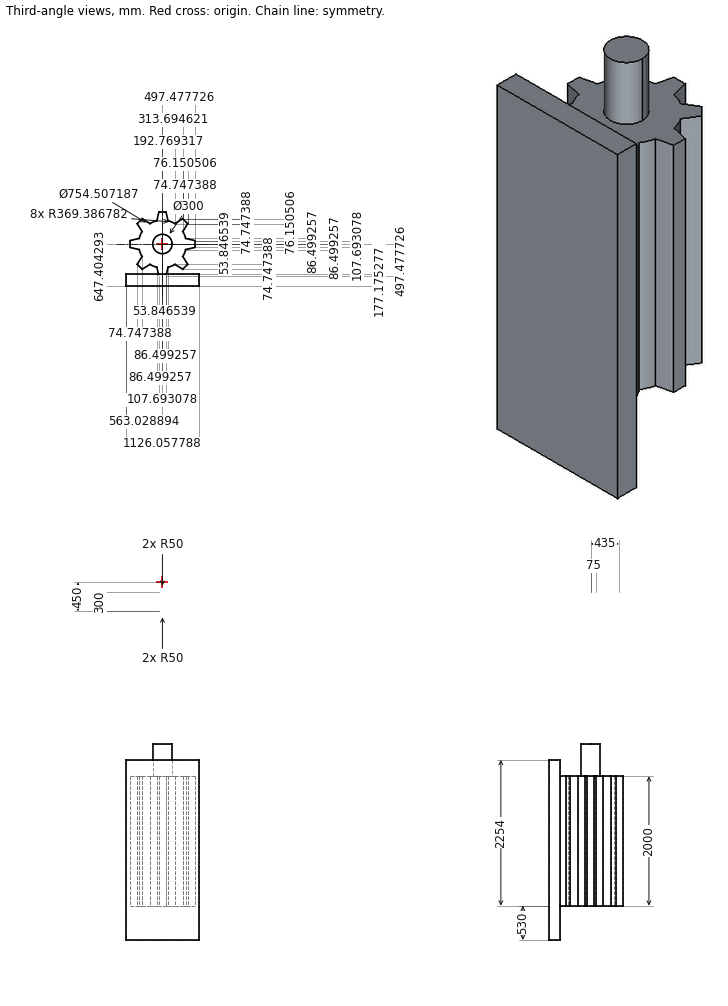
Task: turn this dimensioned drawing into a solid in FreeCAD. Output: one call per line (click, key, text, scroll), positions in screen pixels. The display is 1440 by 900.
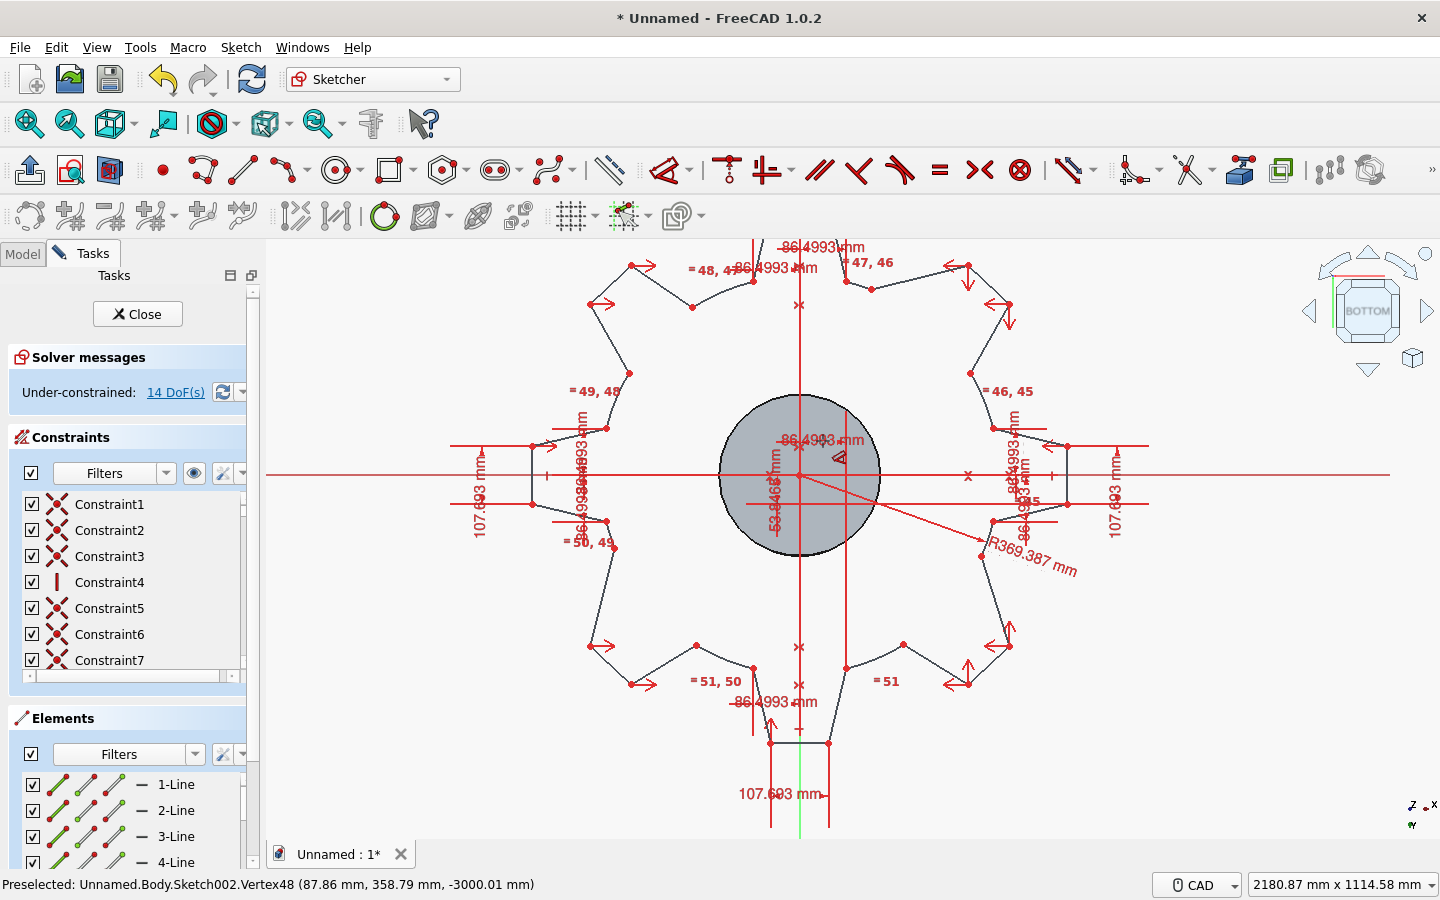
click(923, 657)
click(1002, 674)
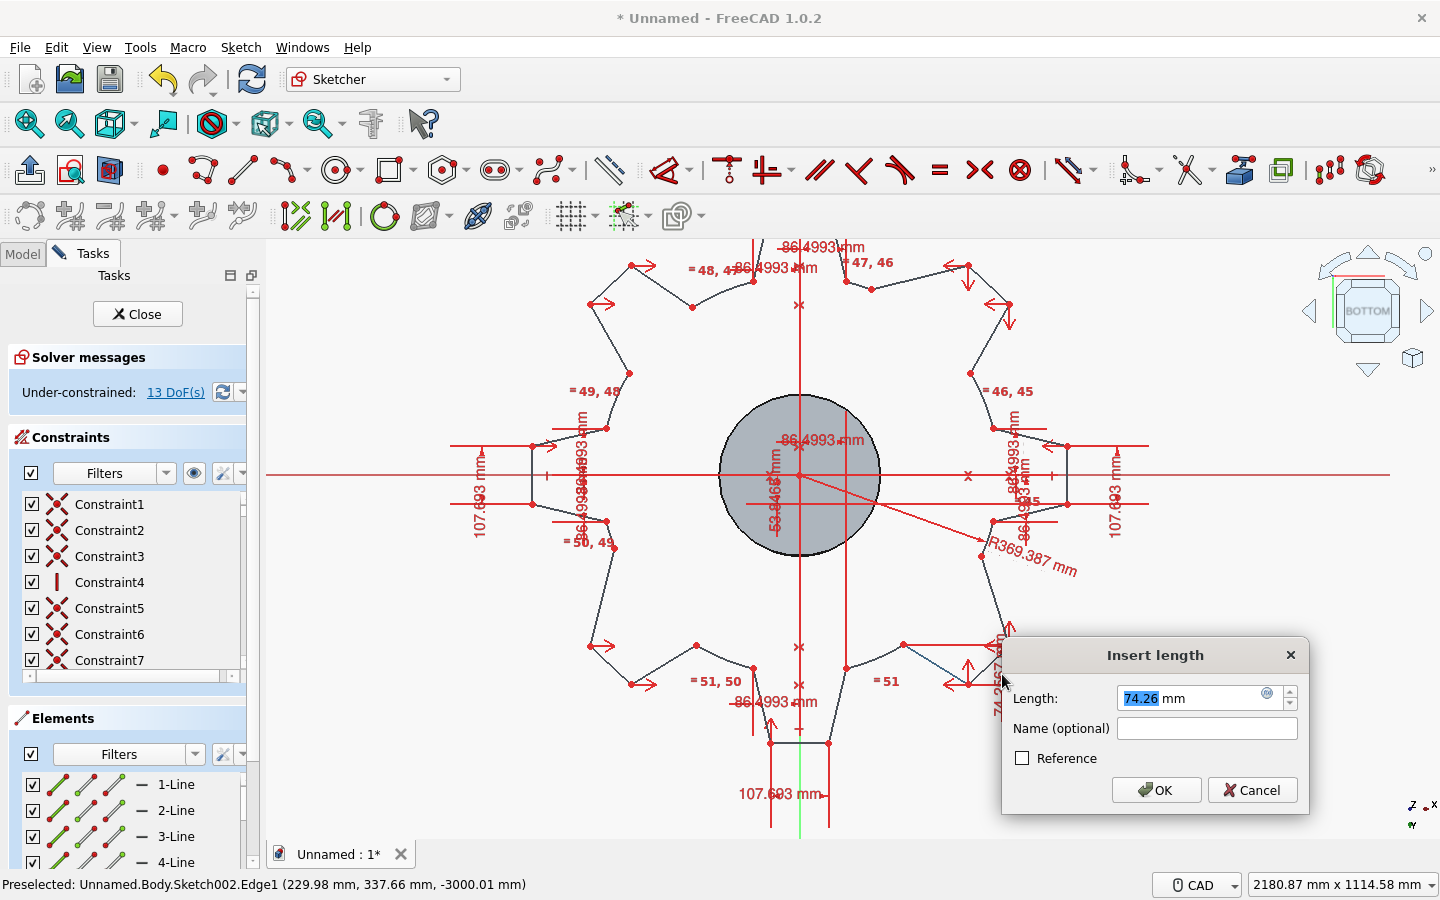
text(74.747388)
key(Return)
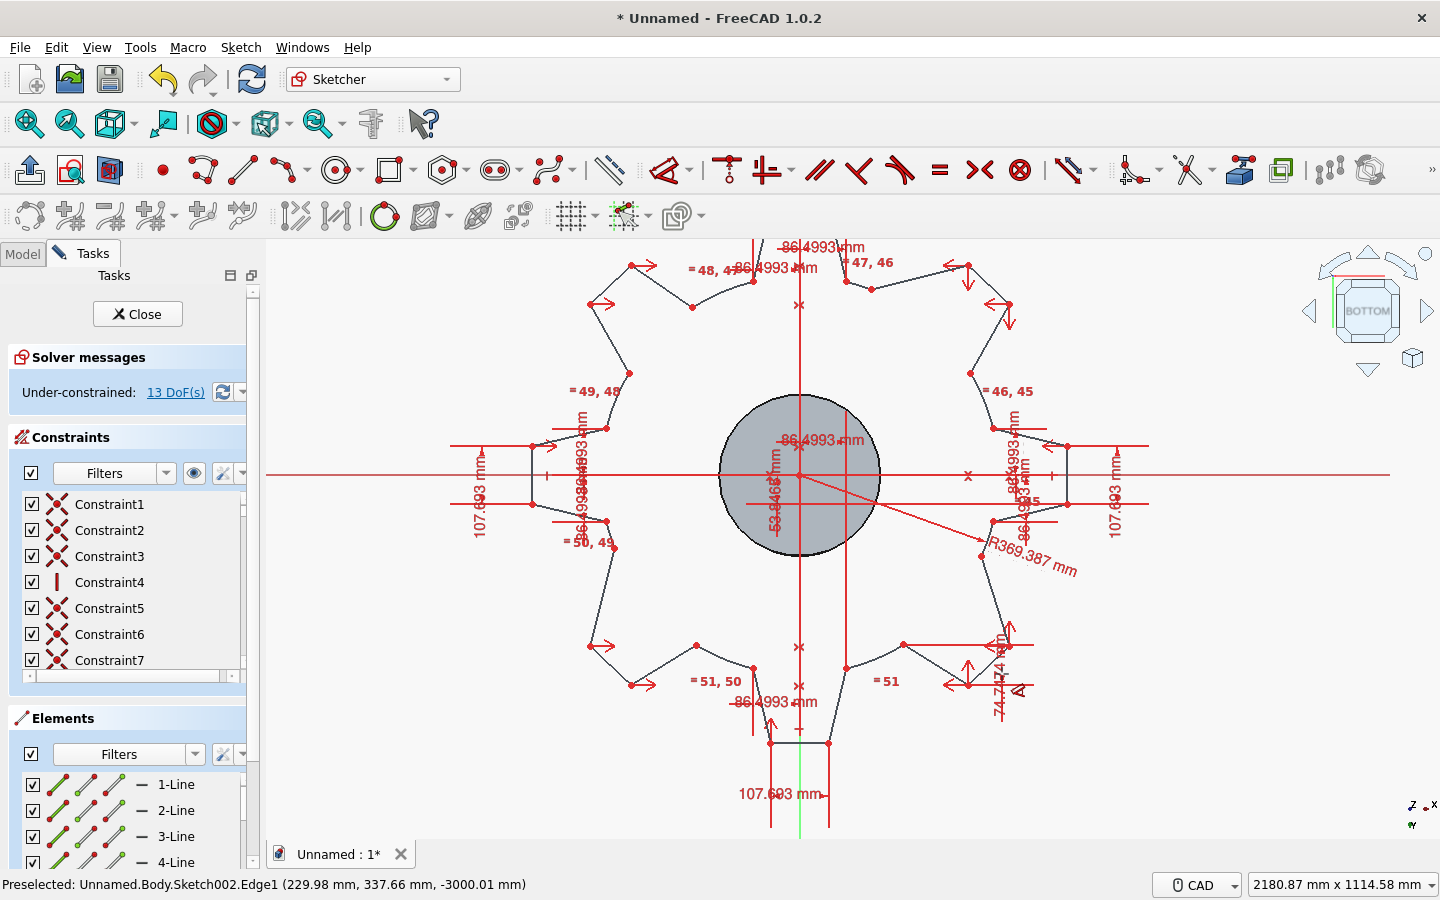
click(981, 673)
click(989, 719)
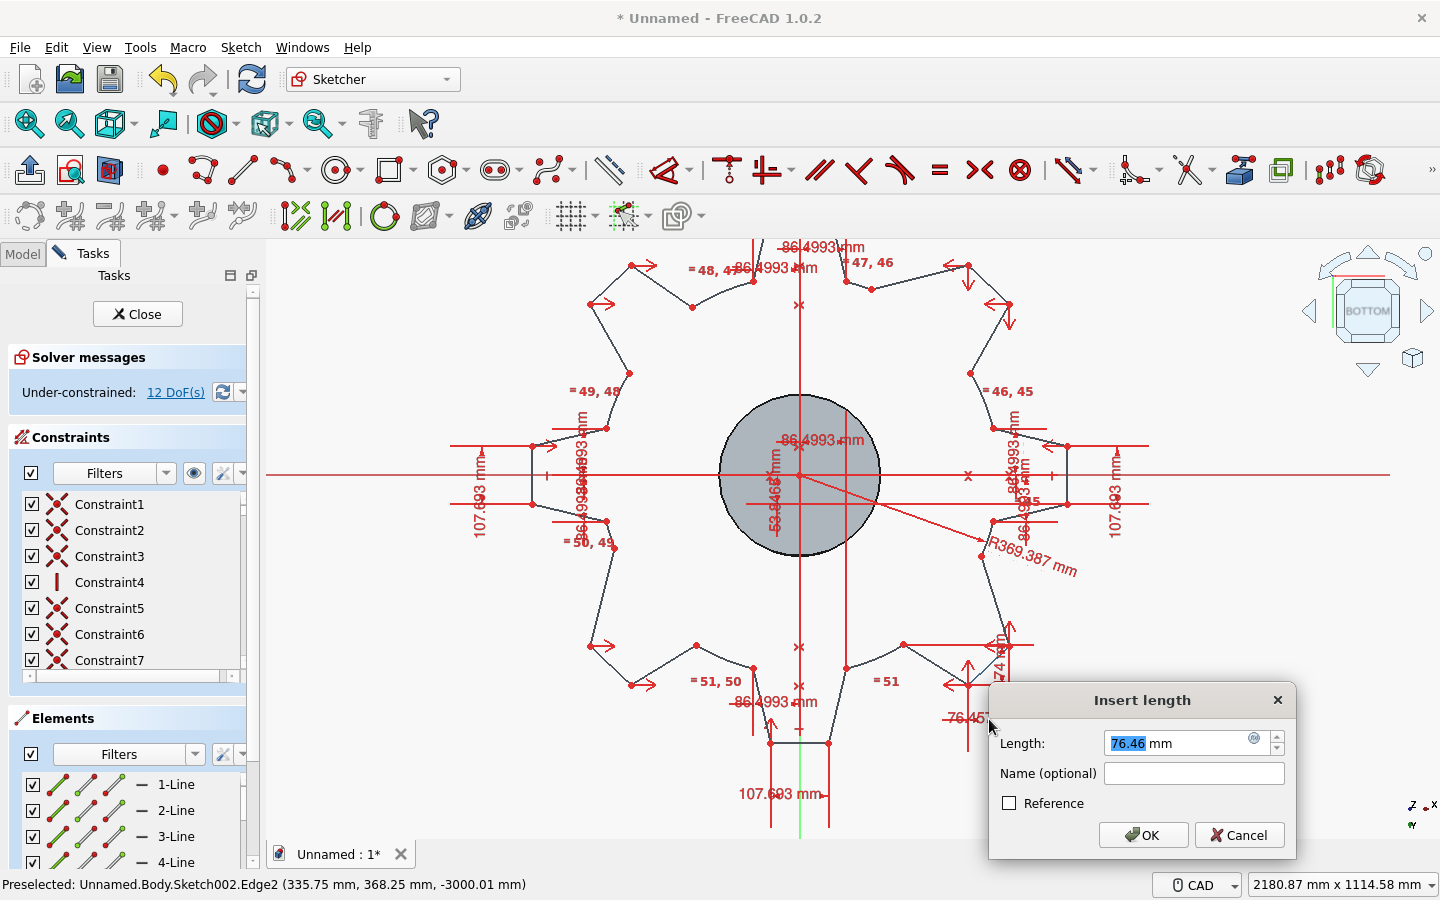
text(76.150506)
key(Return)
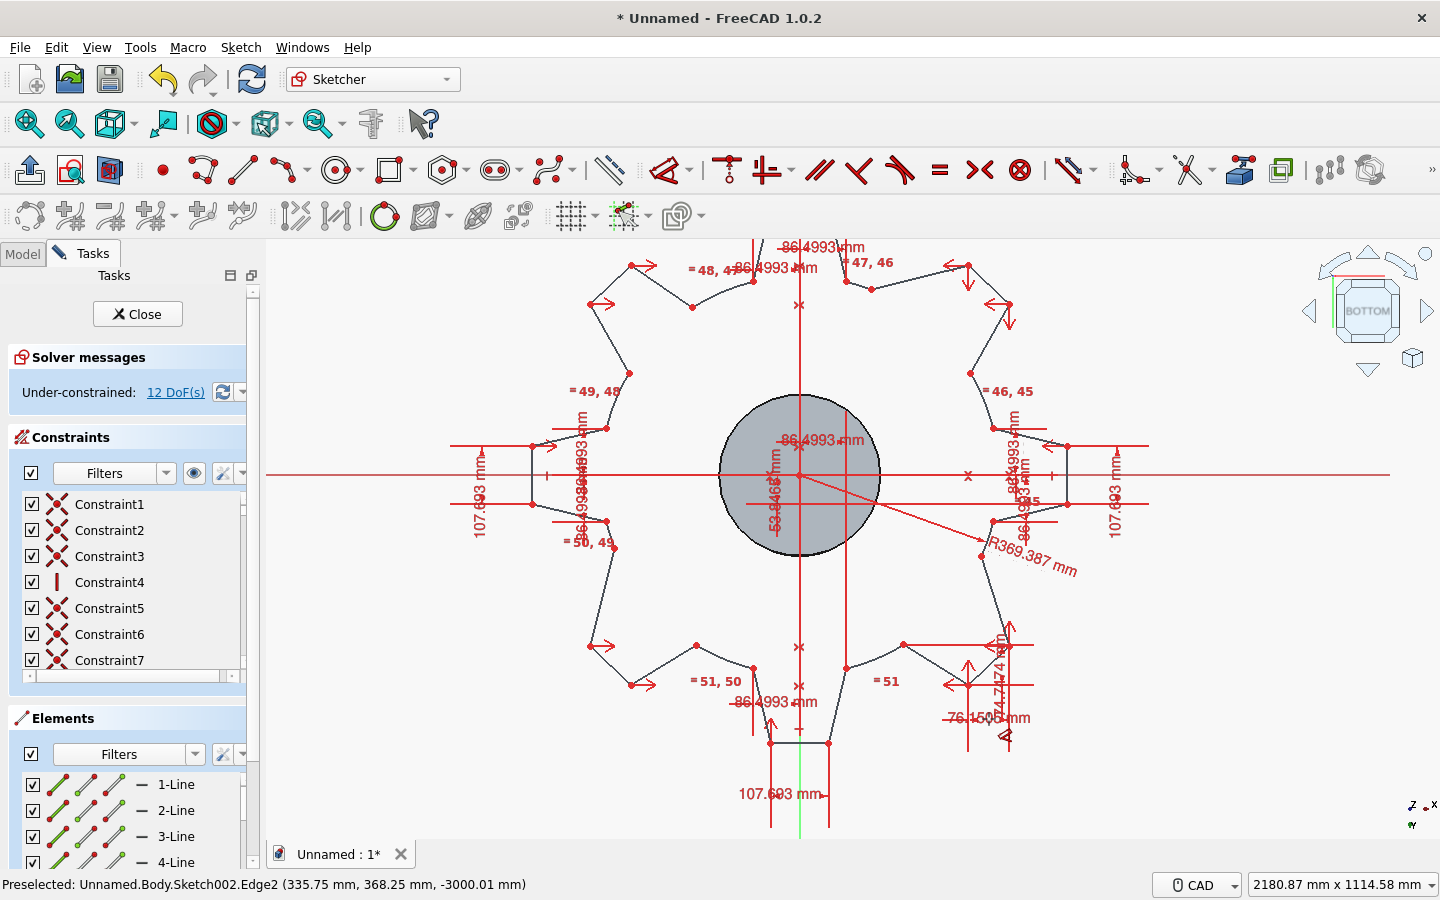
click(981, 673)
click(1043, 652)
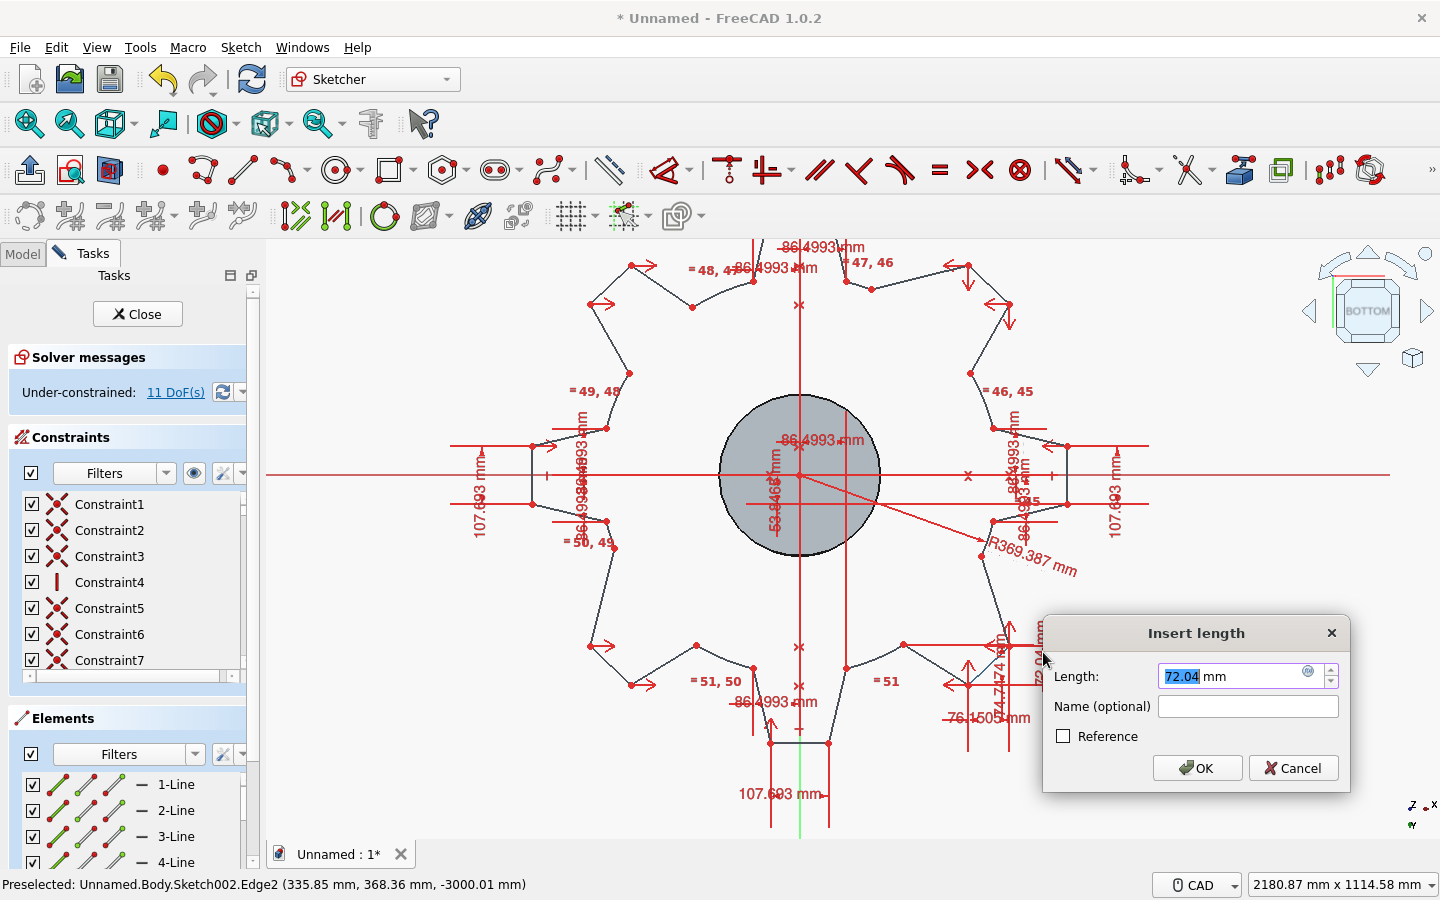
text(76.150506)
key(Return)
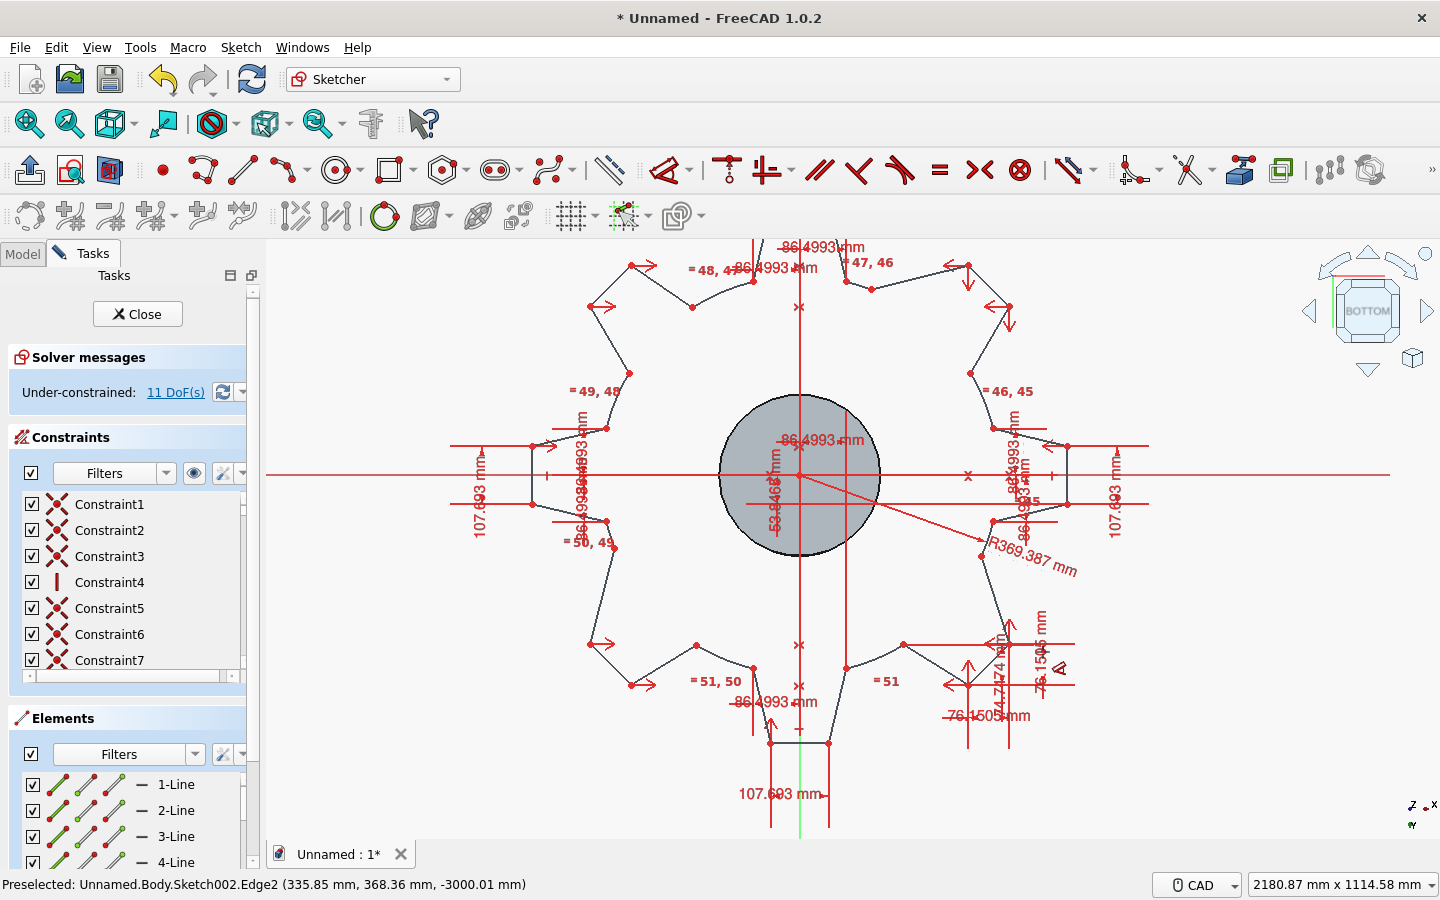
click(1001, 618)
click(995, 750)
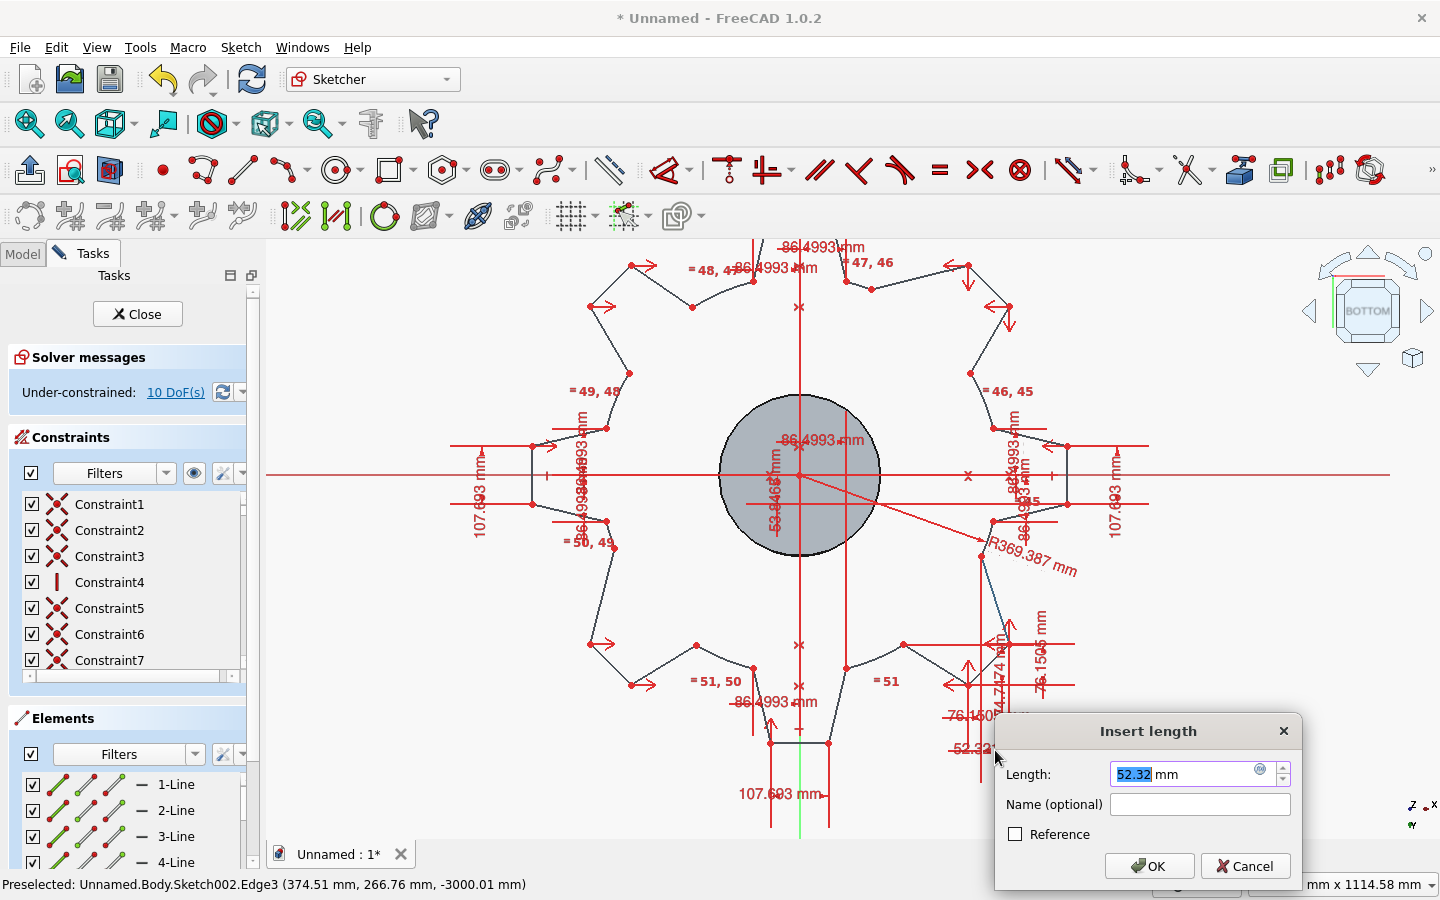
text(74.747388)
key(Return)